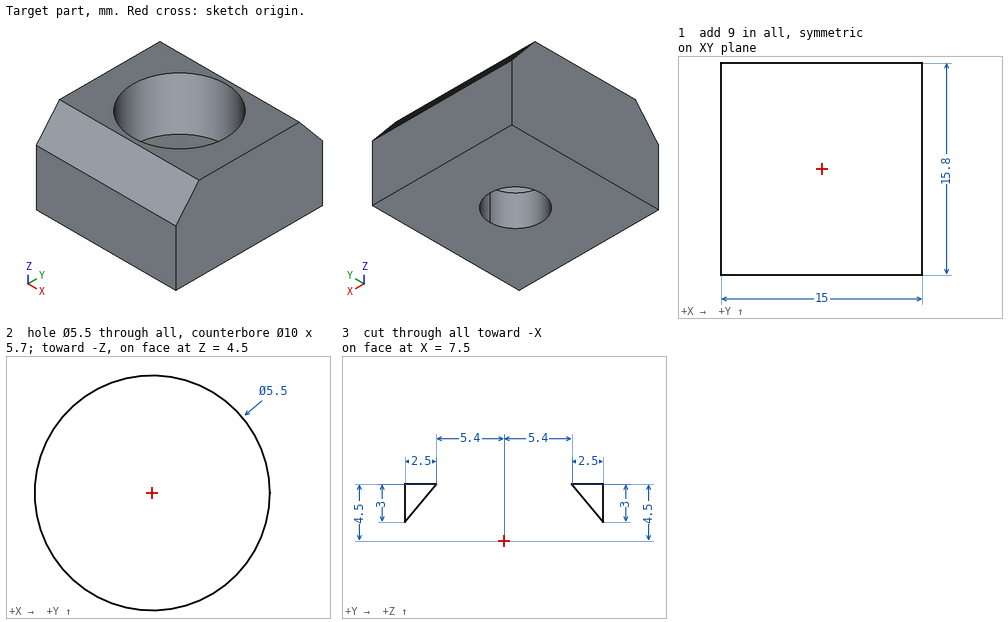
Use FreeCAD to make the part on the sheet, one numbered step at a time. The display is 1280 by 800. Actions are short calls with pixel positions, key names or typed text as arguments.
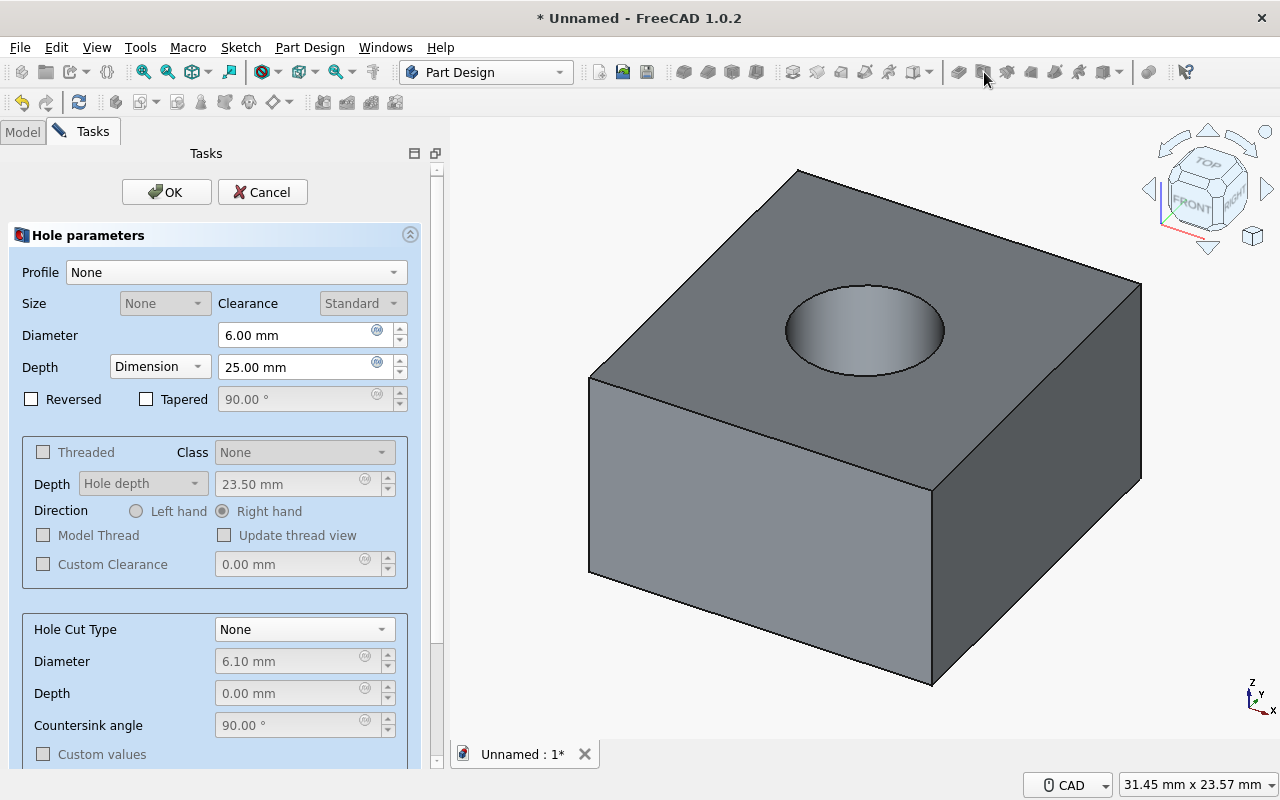
triple_click(305, 335)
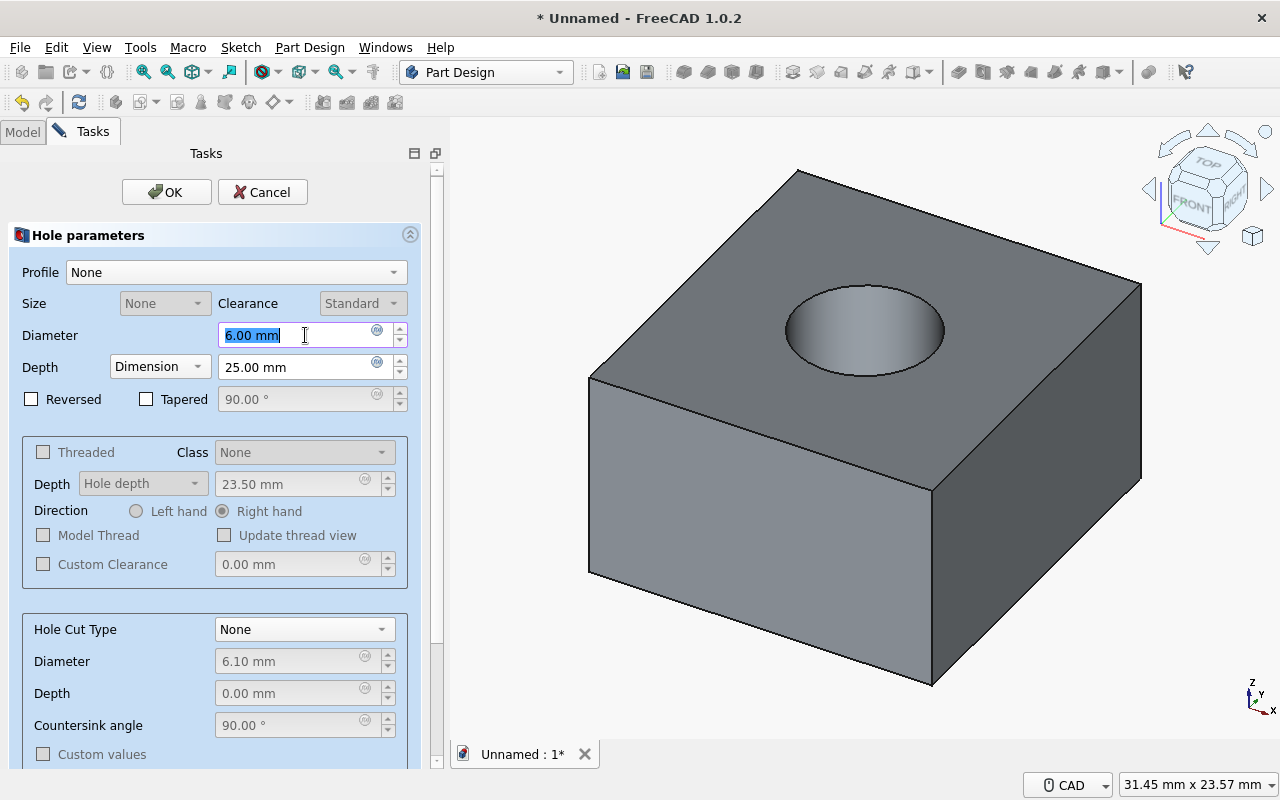
text(5.5)
key(Tab)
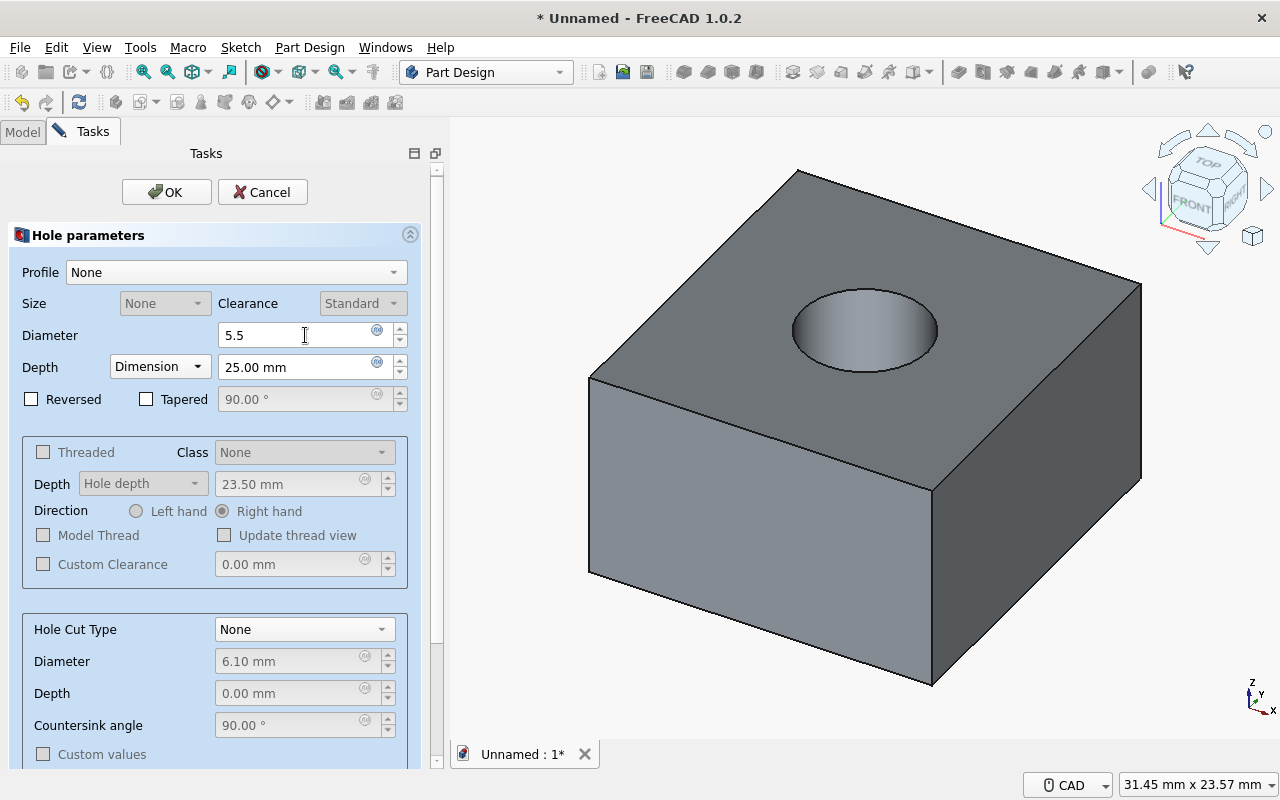
click(161, 366)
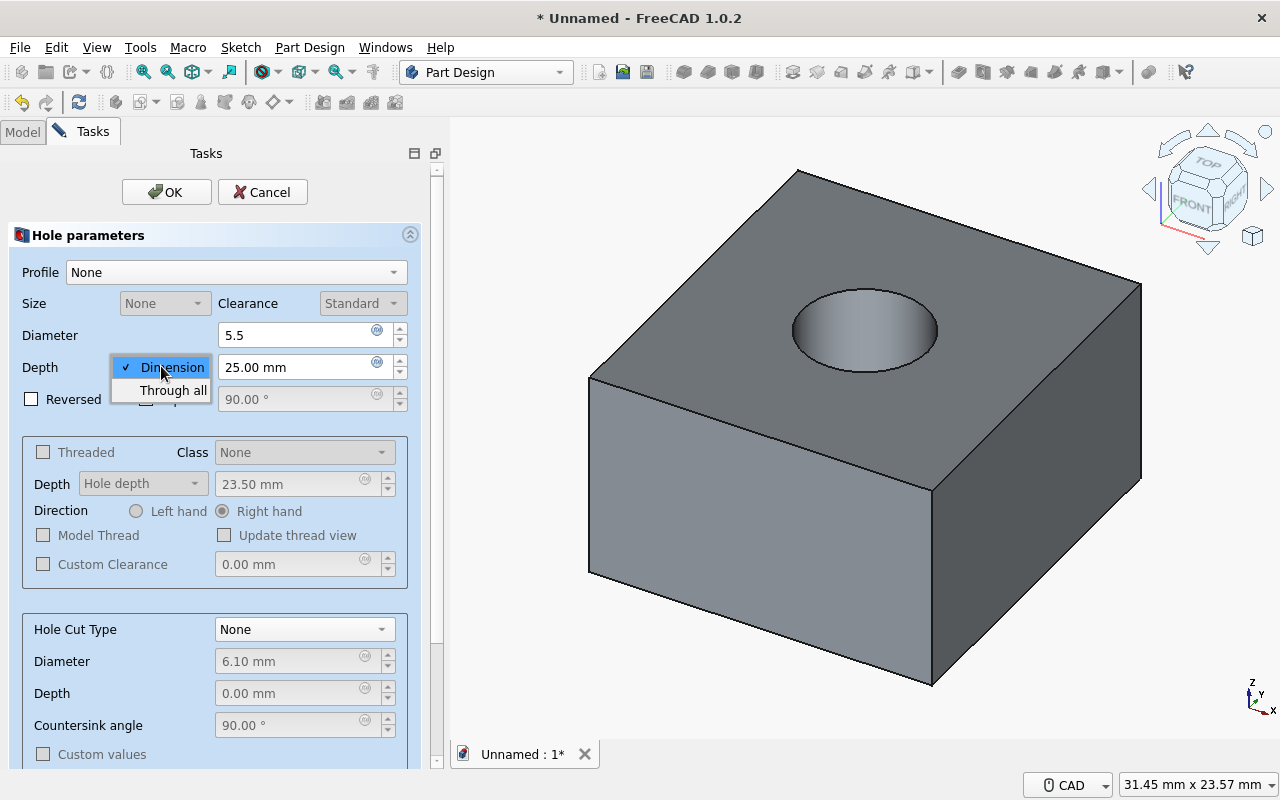
click(160, 390)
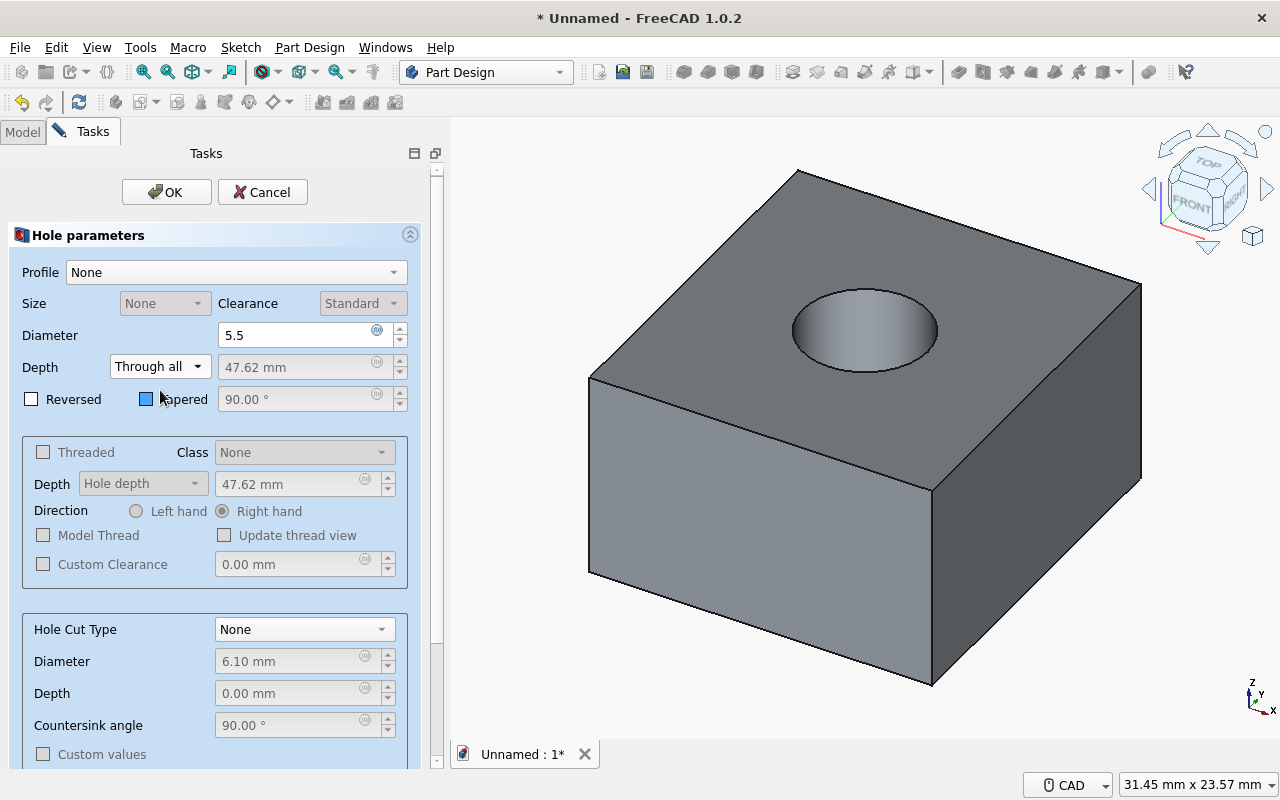
click(306, 630)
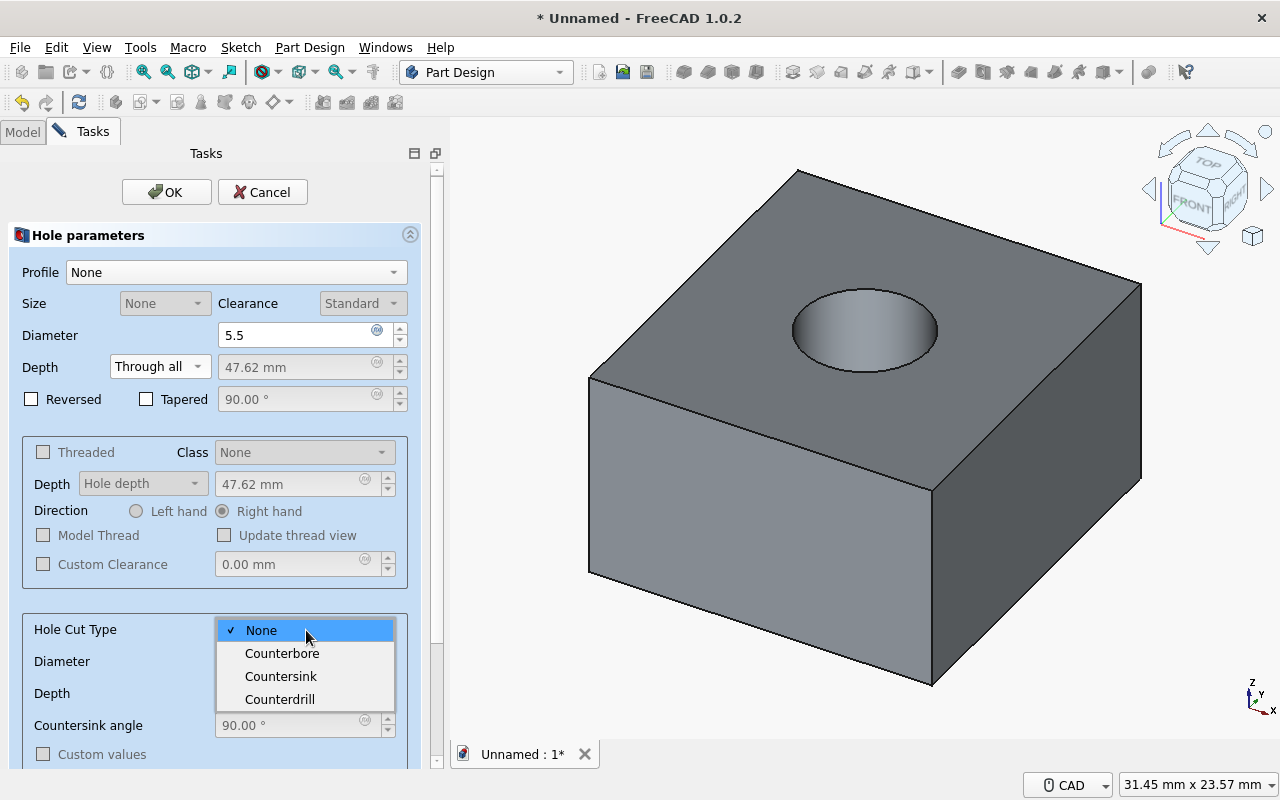
click(304, 654)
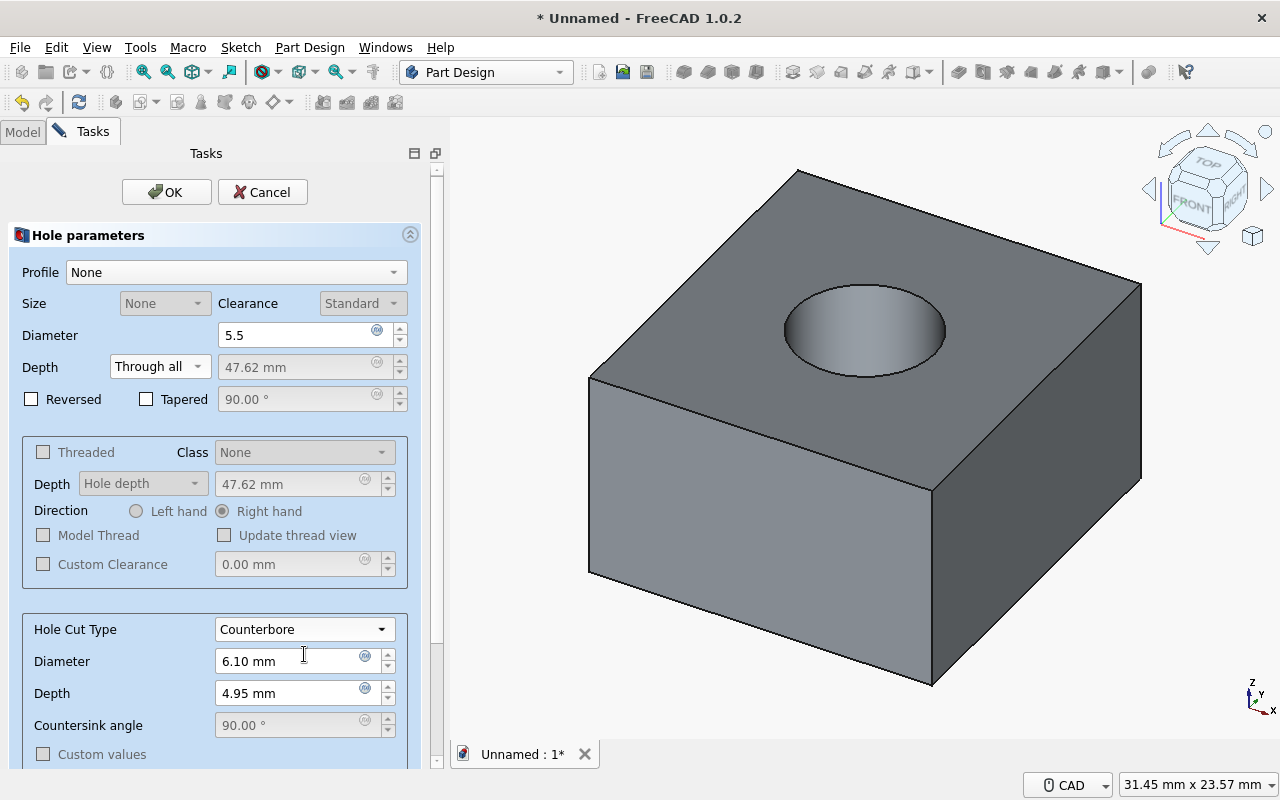
triple_click(298, 661)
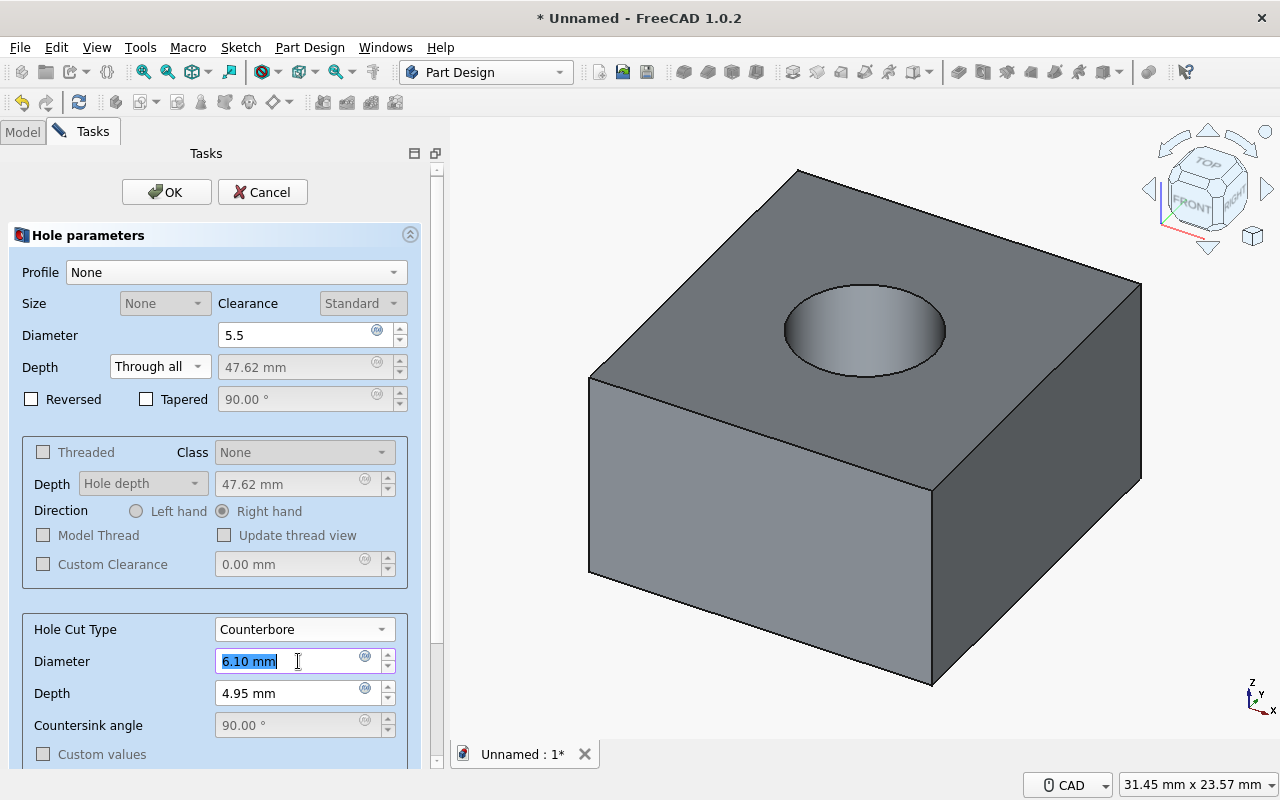
text(10)
key(Tab)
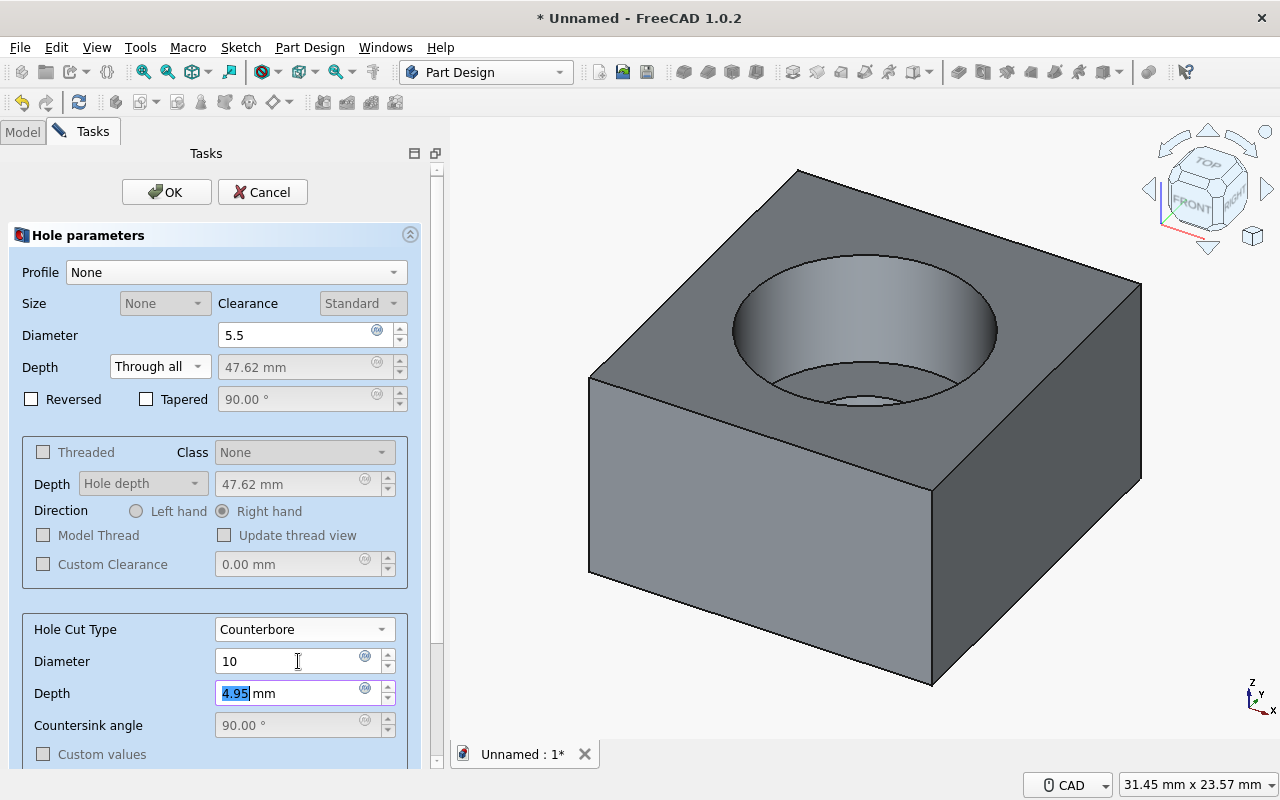
text(5.7)
key(Tab)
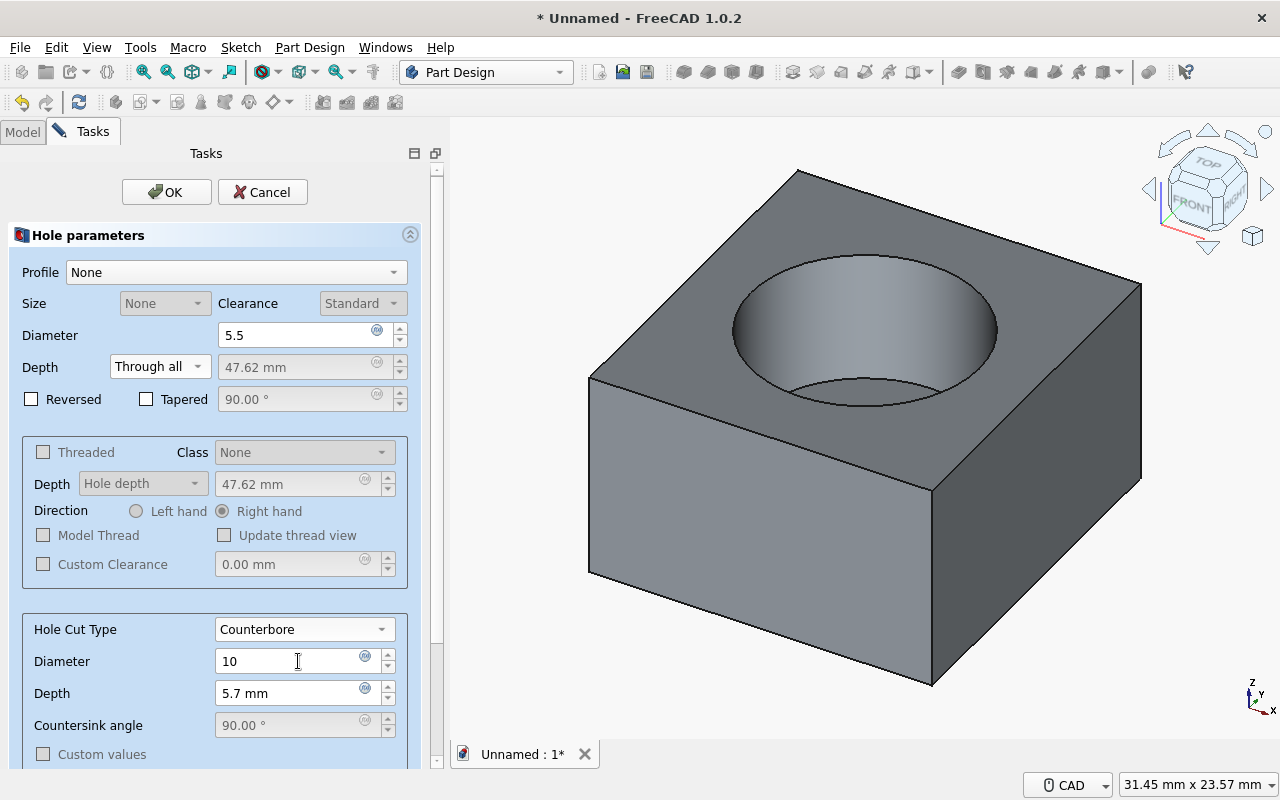
click(167, 192)